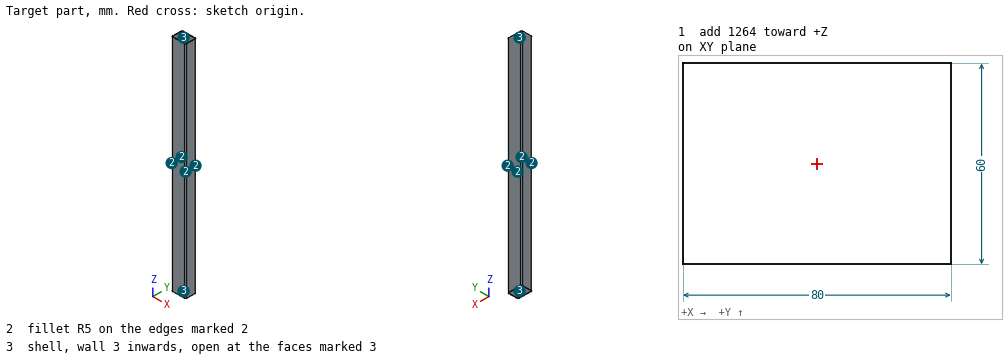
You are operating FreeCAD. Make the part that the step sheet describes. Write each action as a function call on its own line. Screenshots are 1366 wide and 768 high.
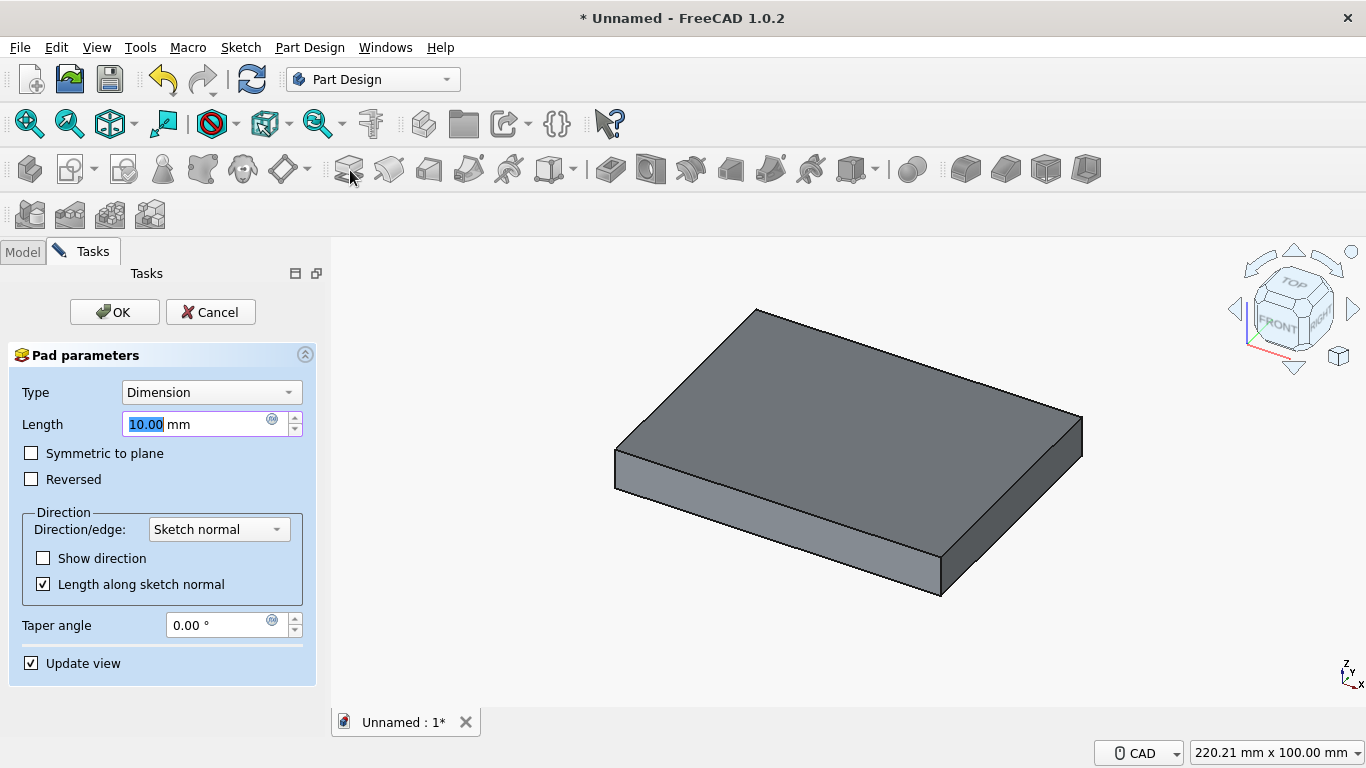
text(1264)
key(Tab)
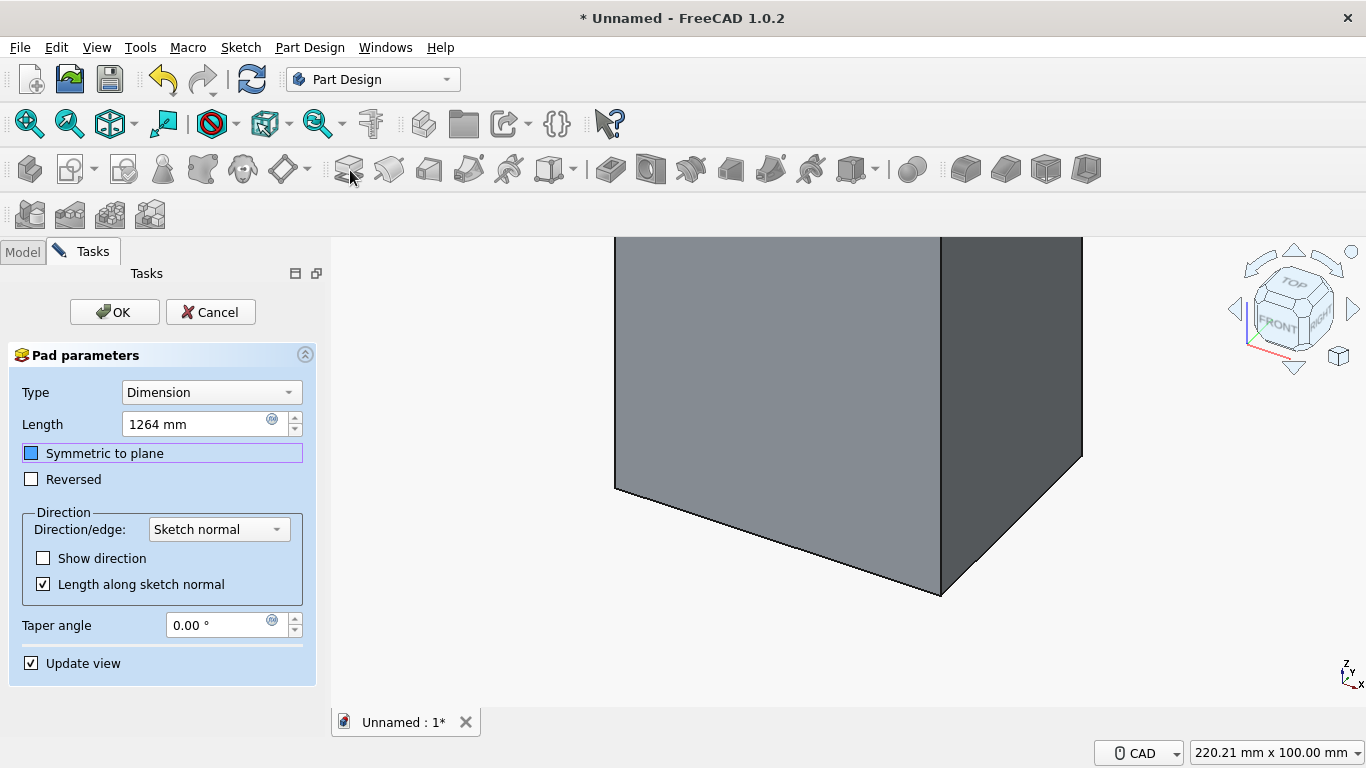
click(115, 312)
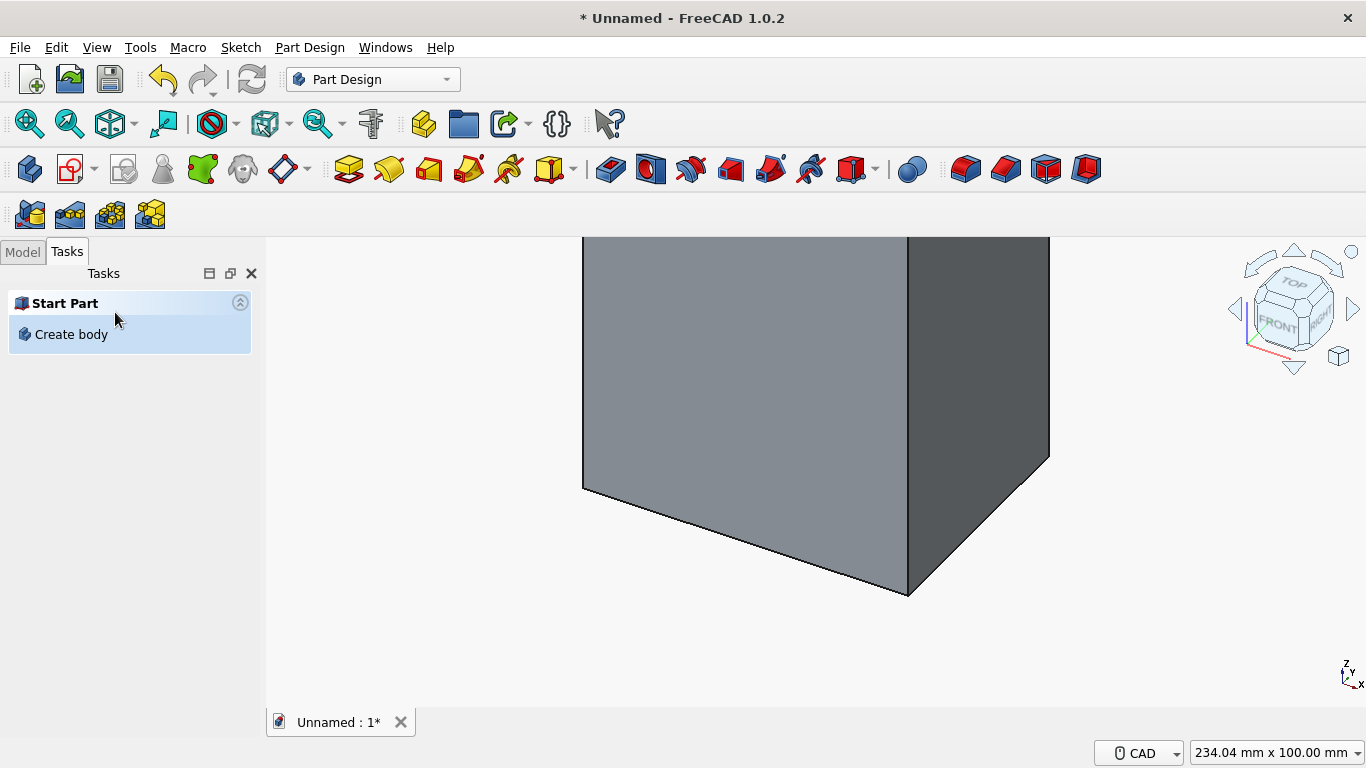
key(v)
key(f)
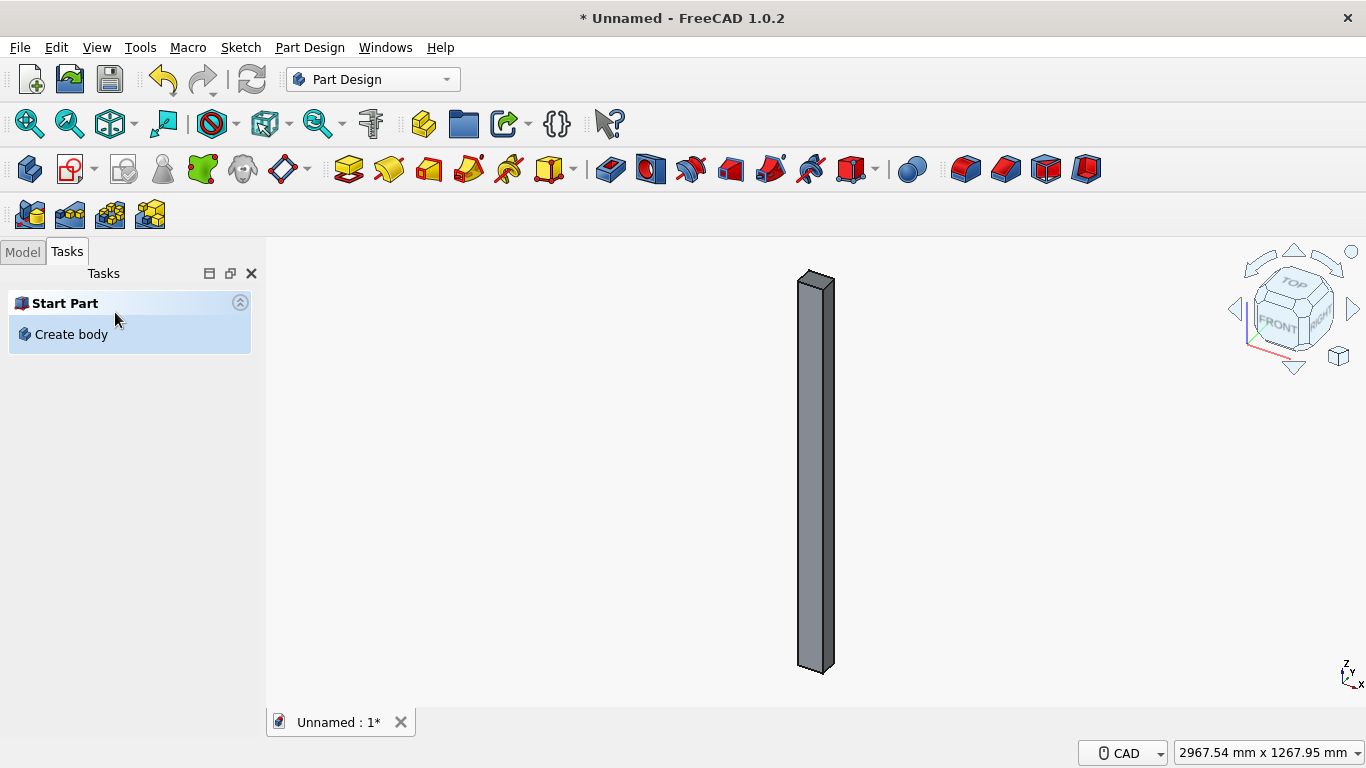
click(823, 481)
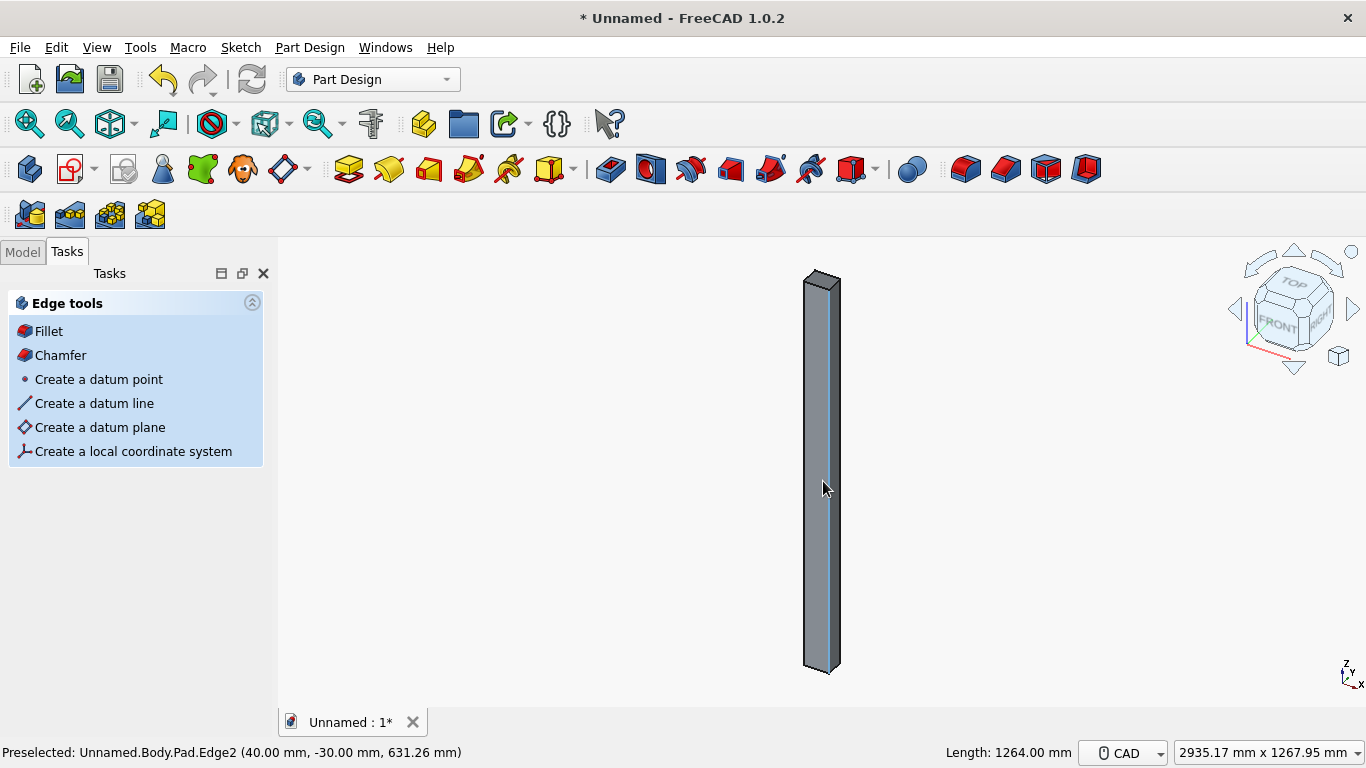
key(0)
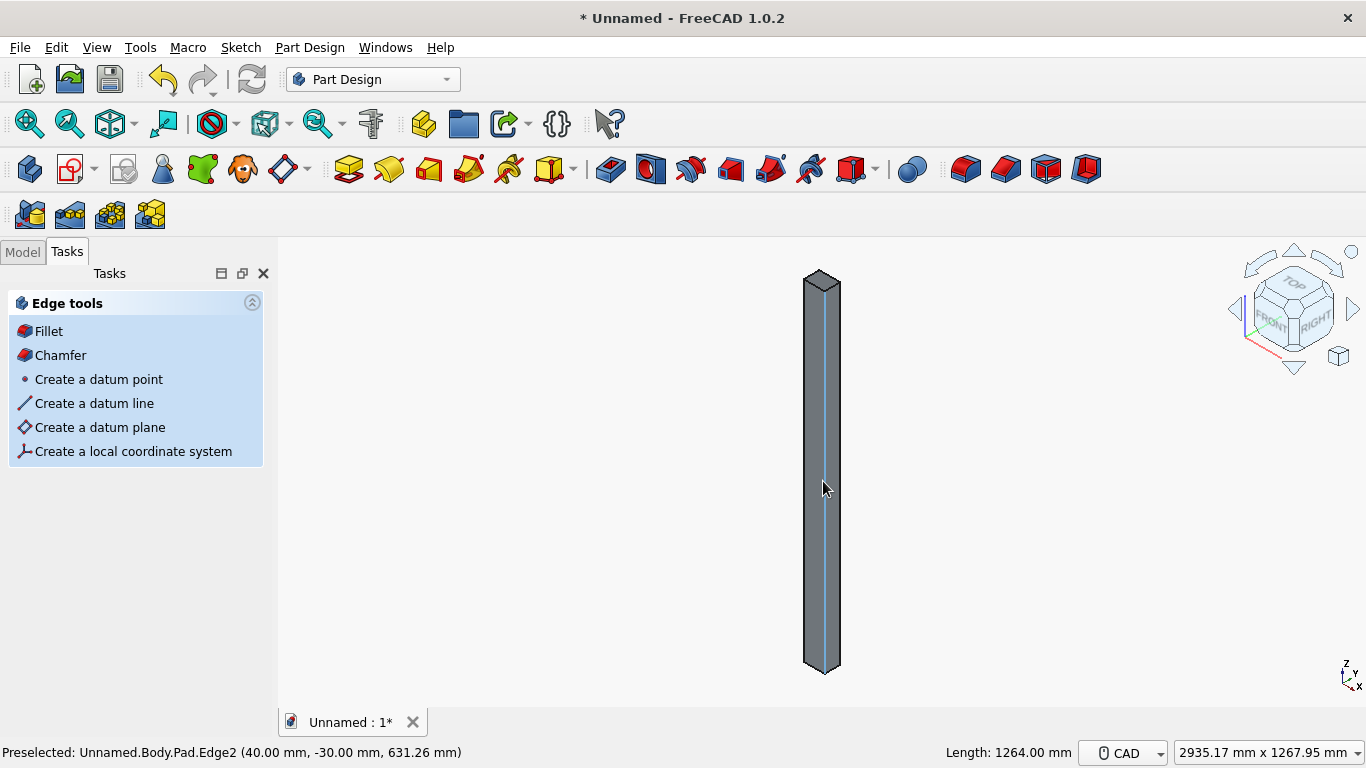
key(2)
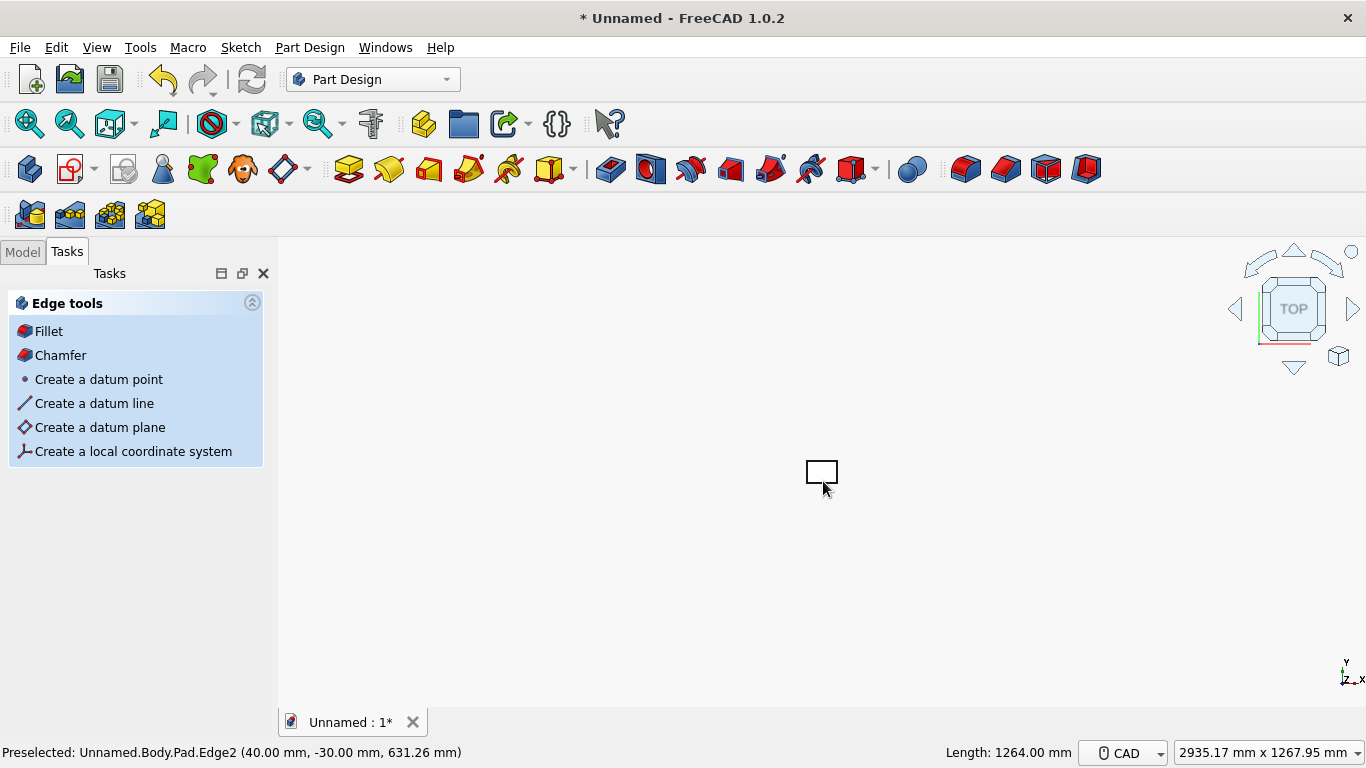
key(v)
key(f)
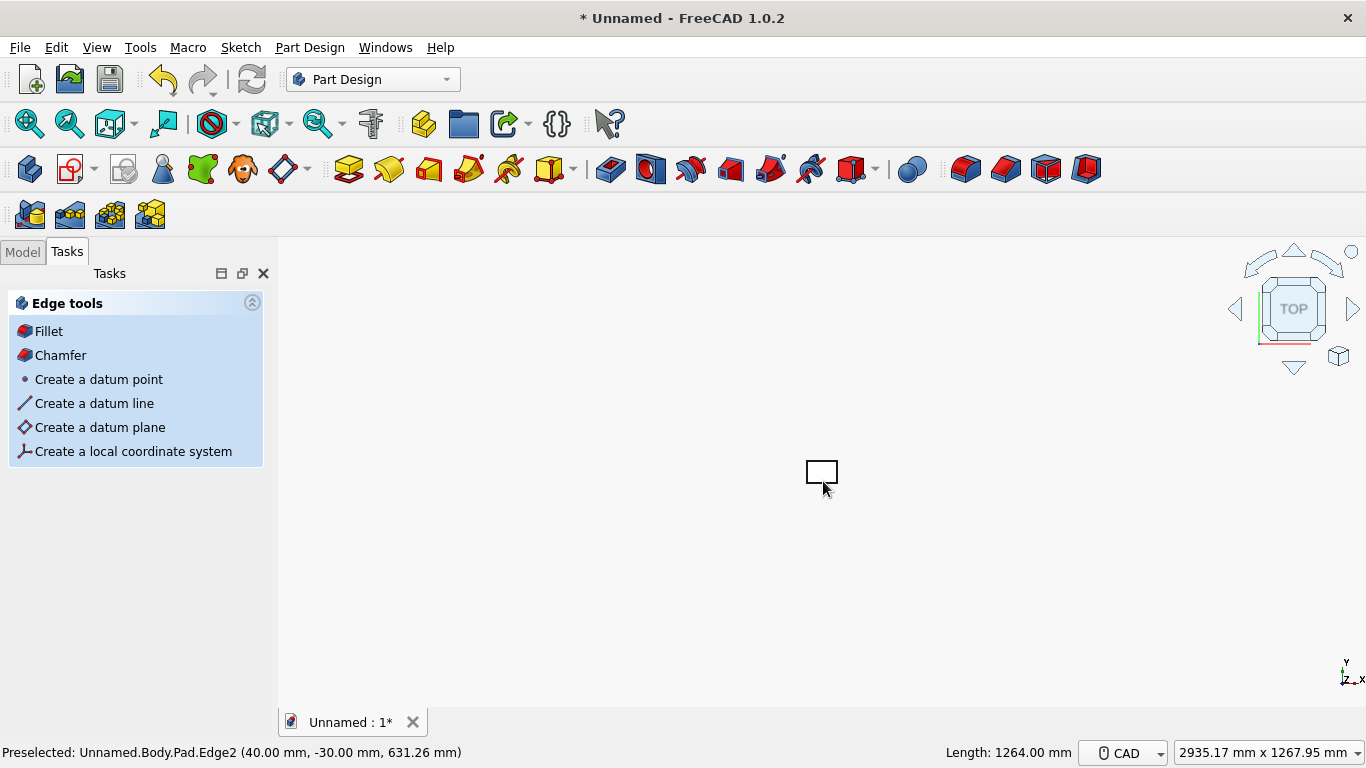
key(1)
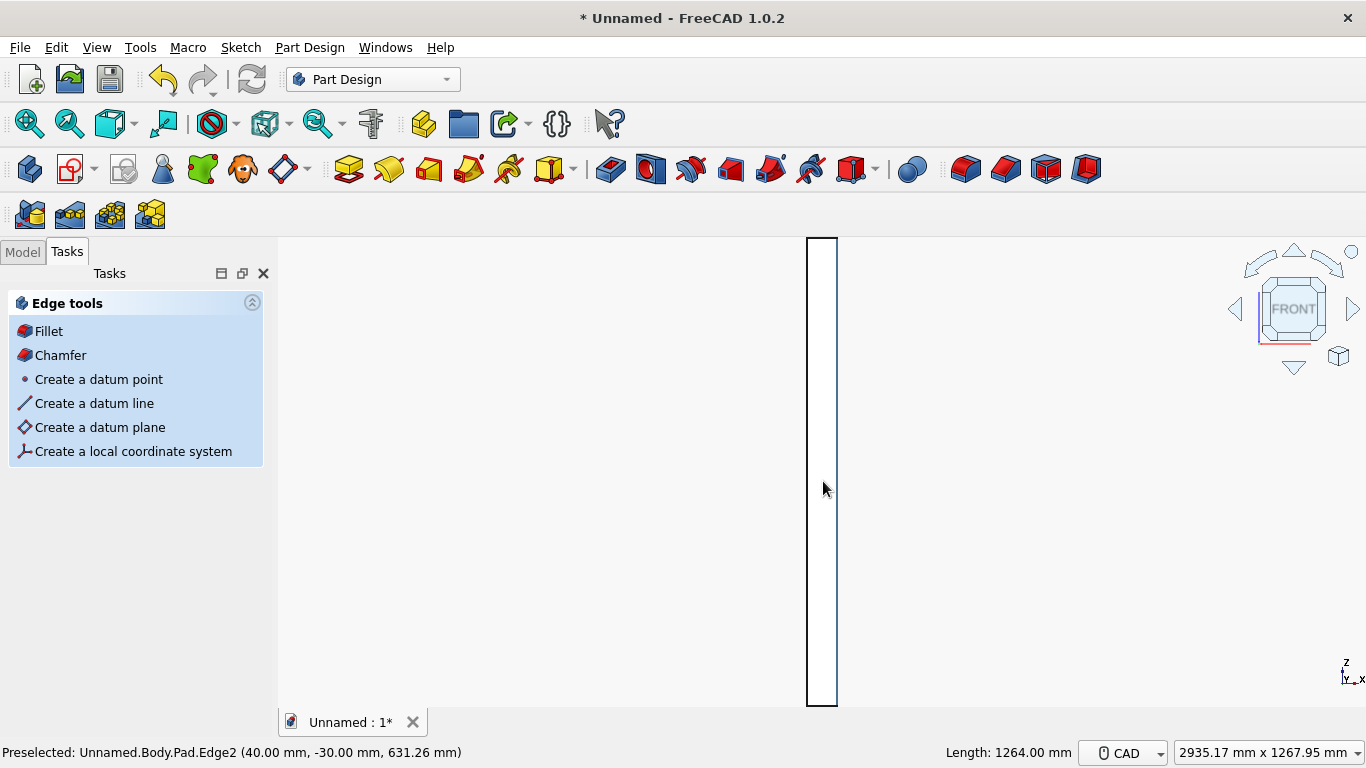
click(807, 471, ctrl)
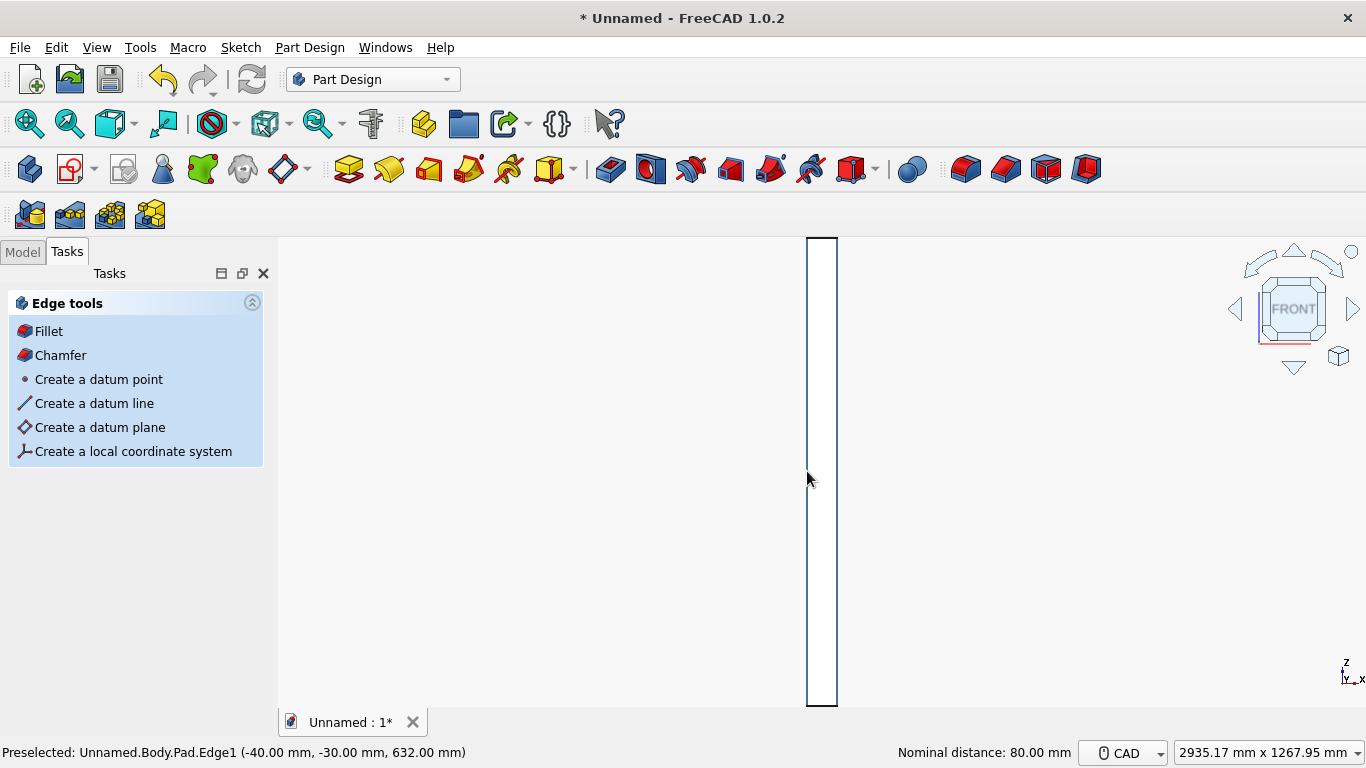
key(3)